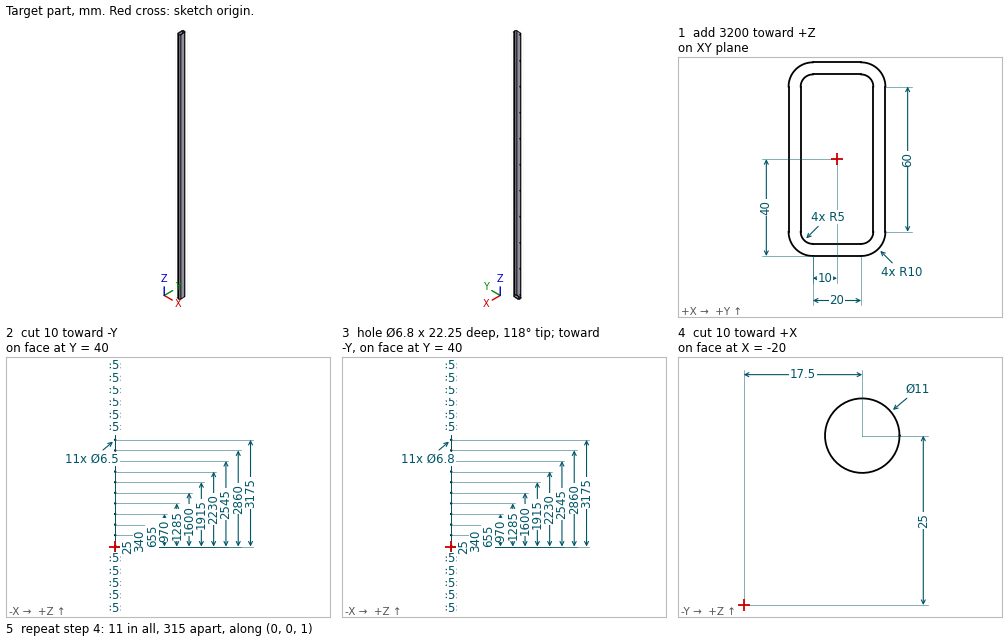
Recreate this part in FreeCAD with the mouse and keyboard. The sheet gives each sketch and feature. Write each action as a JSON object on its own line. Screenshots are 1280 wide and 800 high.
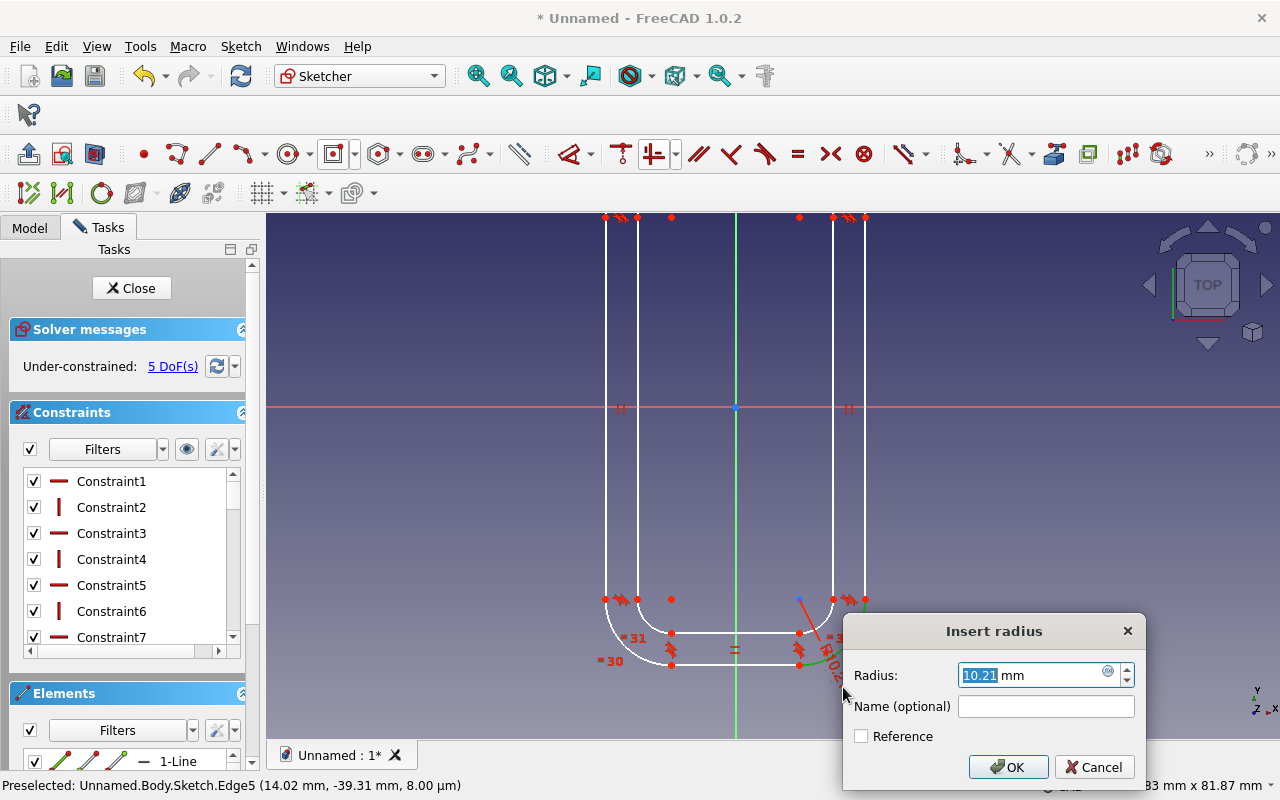
{"action": "type", "text": "10"}
{"action": "key", "text": "Return"}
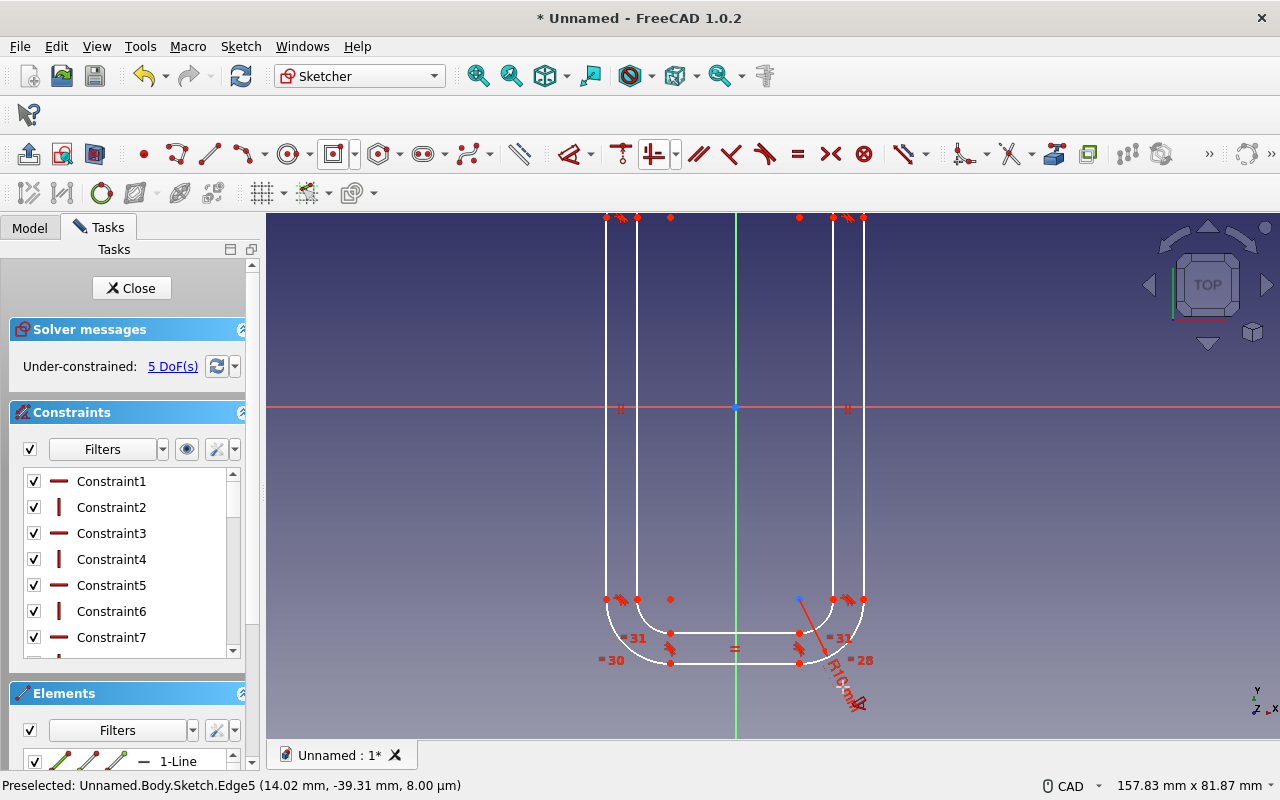
{"action": "scroll", "coordinate": [641, 615], "scroll_direction": "up", "scroll_amount": 2}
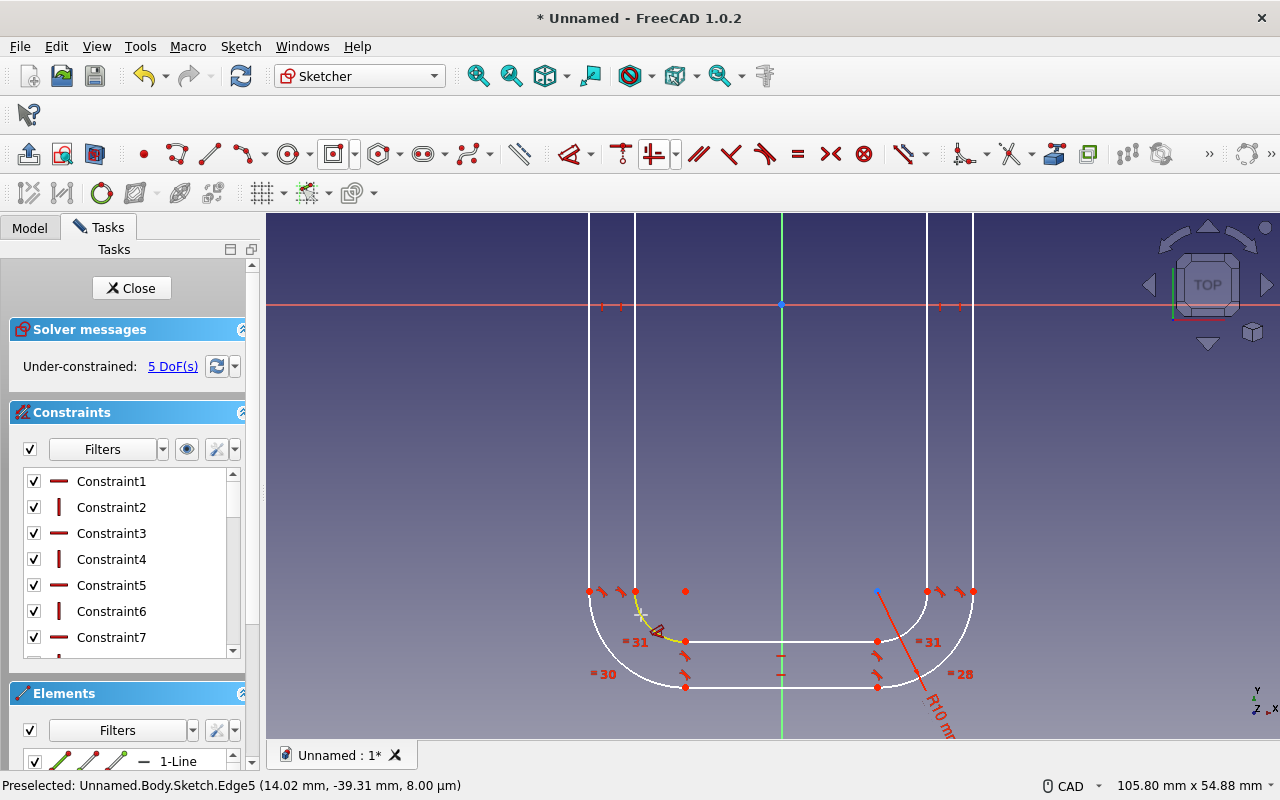
{"action": "left_click", "coordinate": [640, 615]}
{"action": "left_click", "coordinate": [612, 630]}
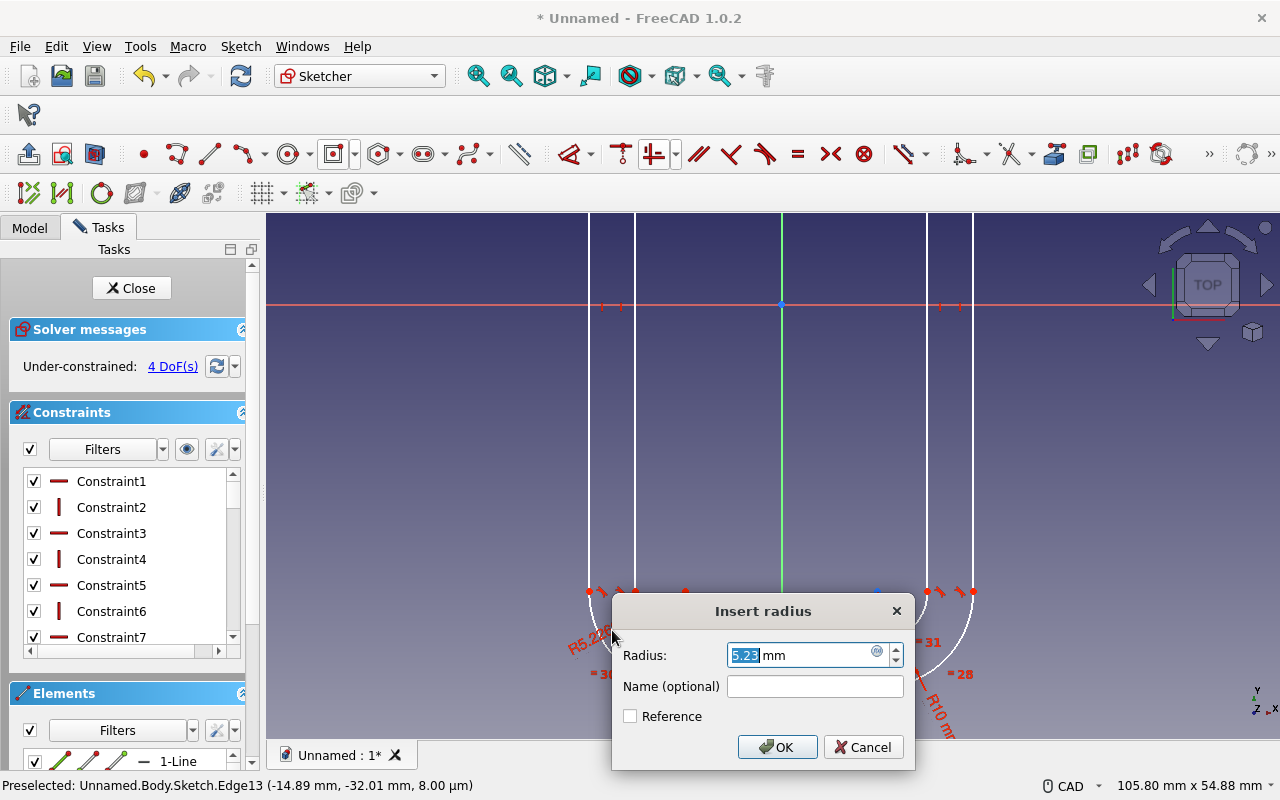
{"action": "type", "text": "5"}
{"action": "key", "text": "Return"}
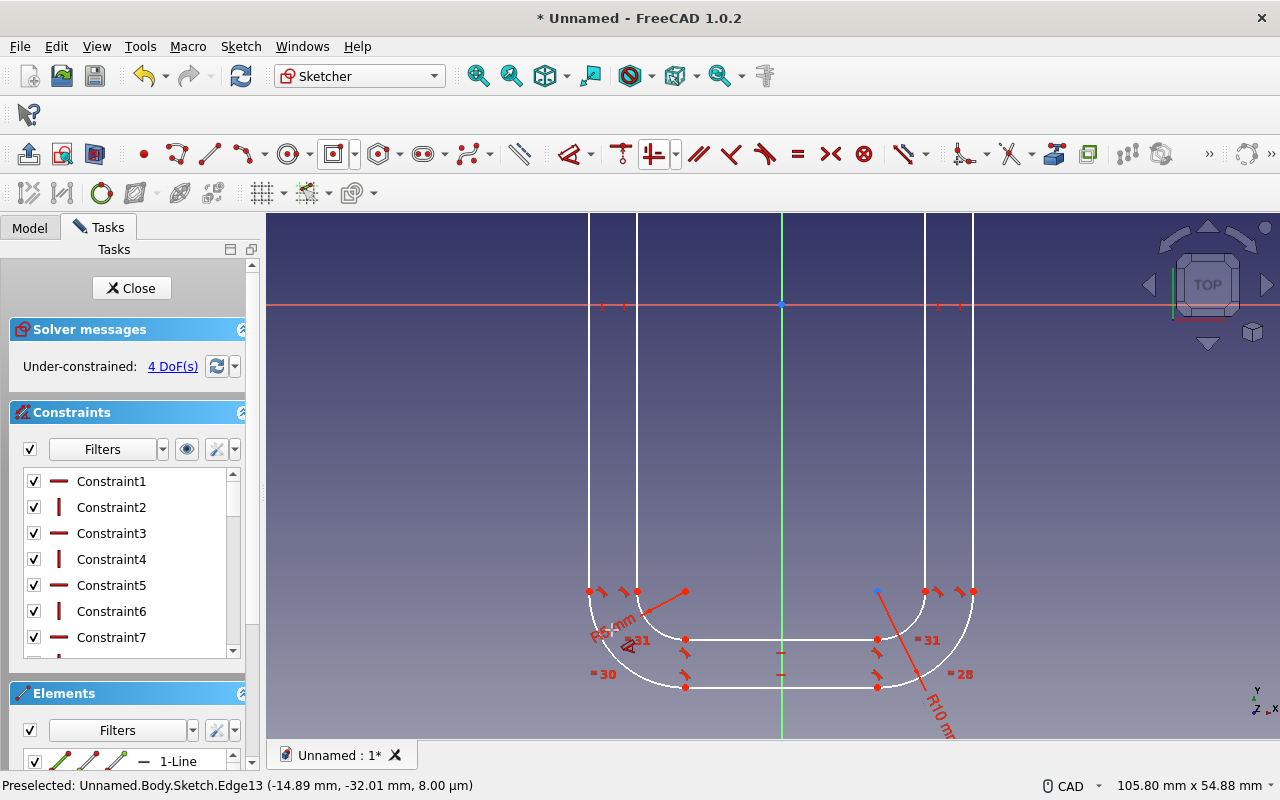
{"action": "left_click", "coordinate": [743, 688]}
{"action": "left_click", "coordinate": [737, 654]}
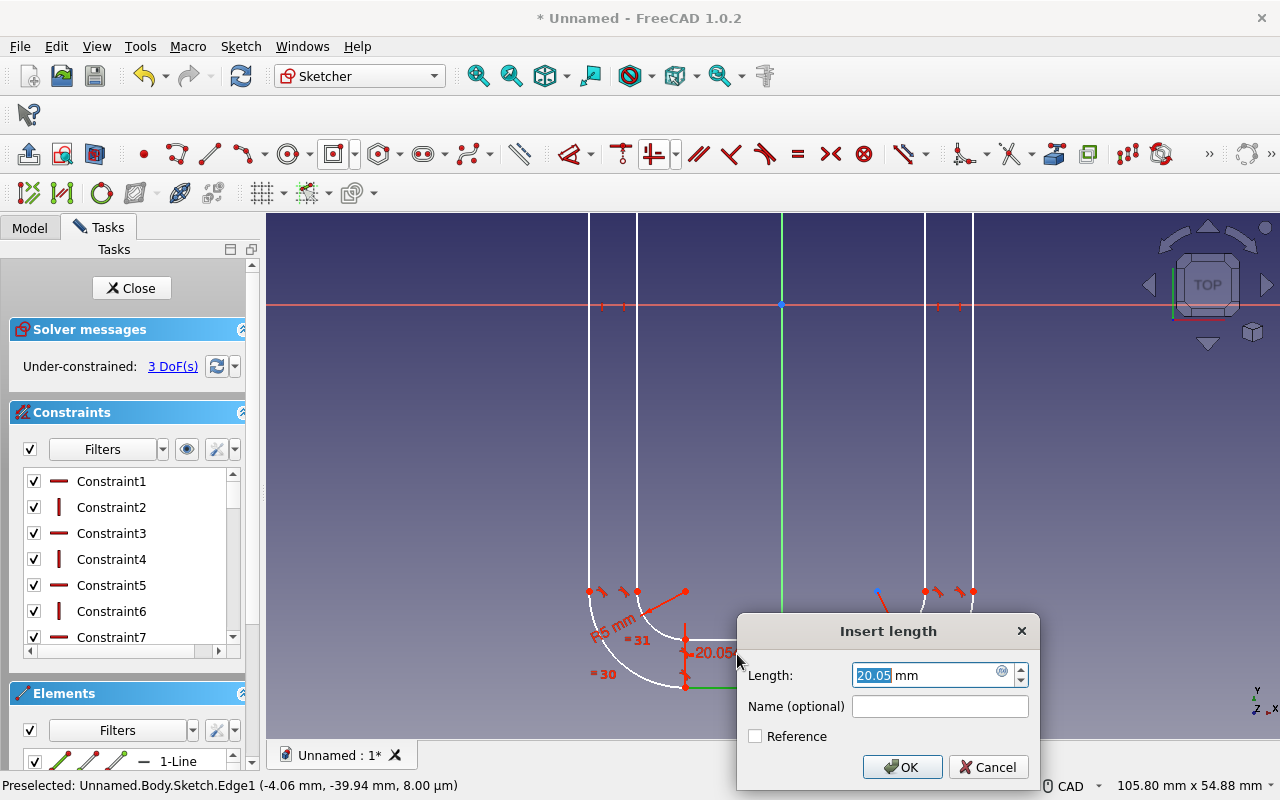
{"action": "type", "text": "20"}
{"action": "key", "text": "Return"}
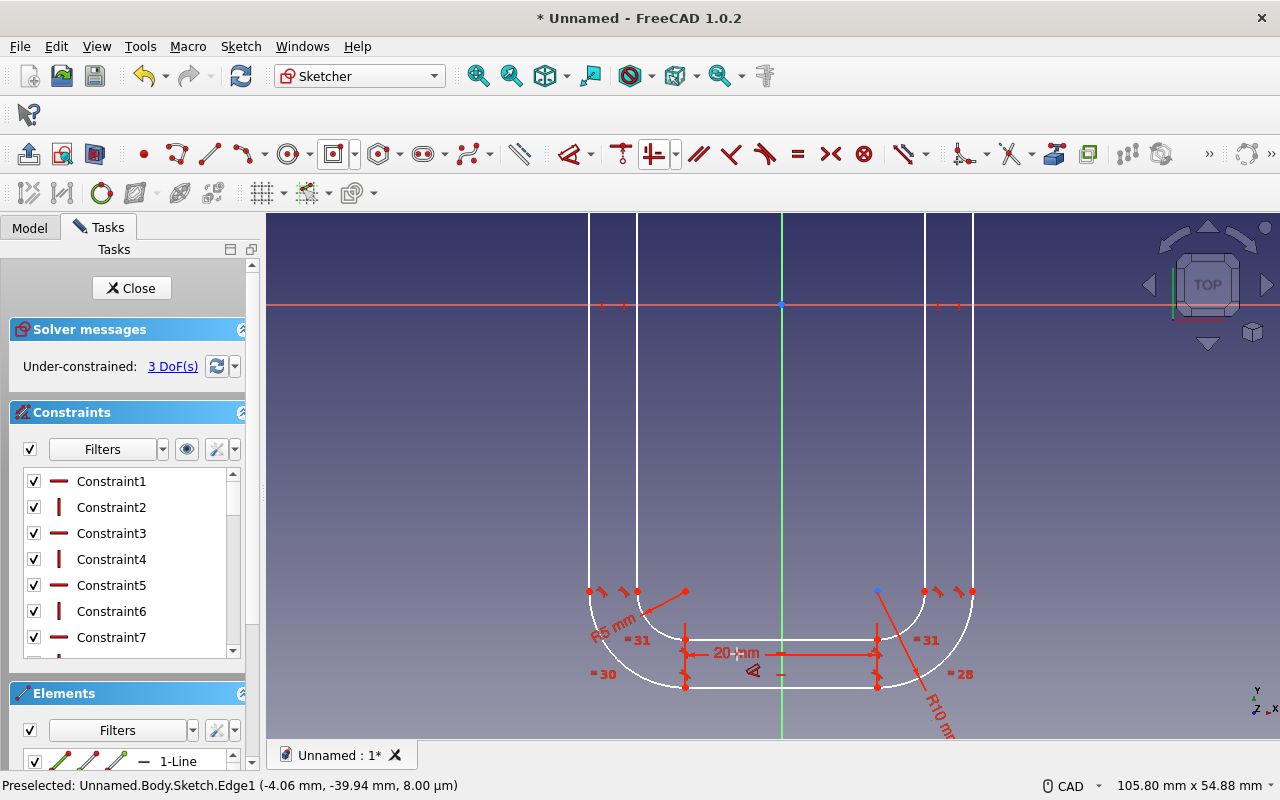
{"action": "left_click", "coordinate": [973, 421]}
{"action": "left_click", "coordinate": [1007, 416]}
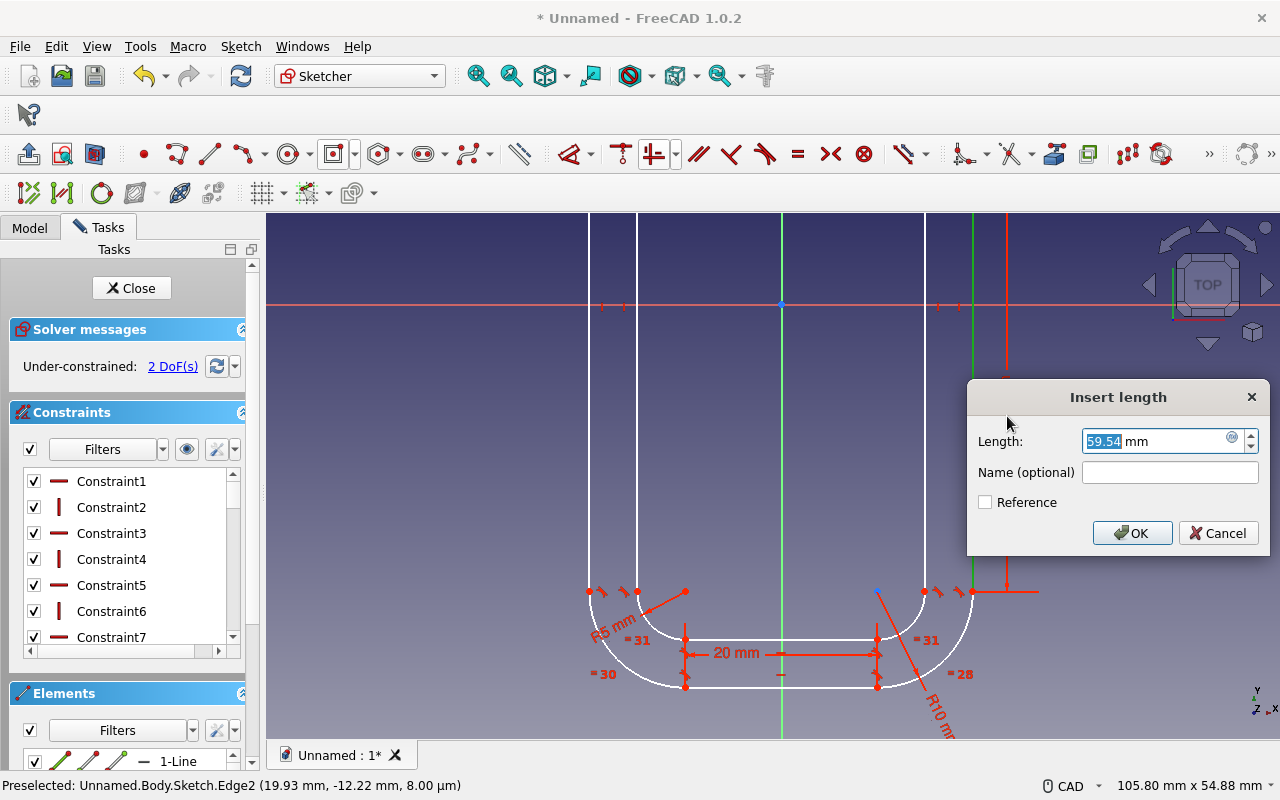
{"action": "type", "text": "60"}
{"action": "key", "text": "Return"}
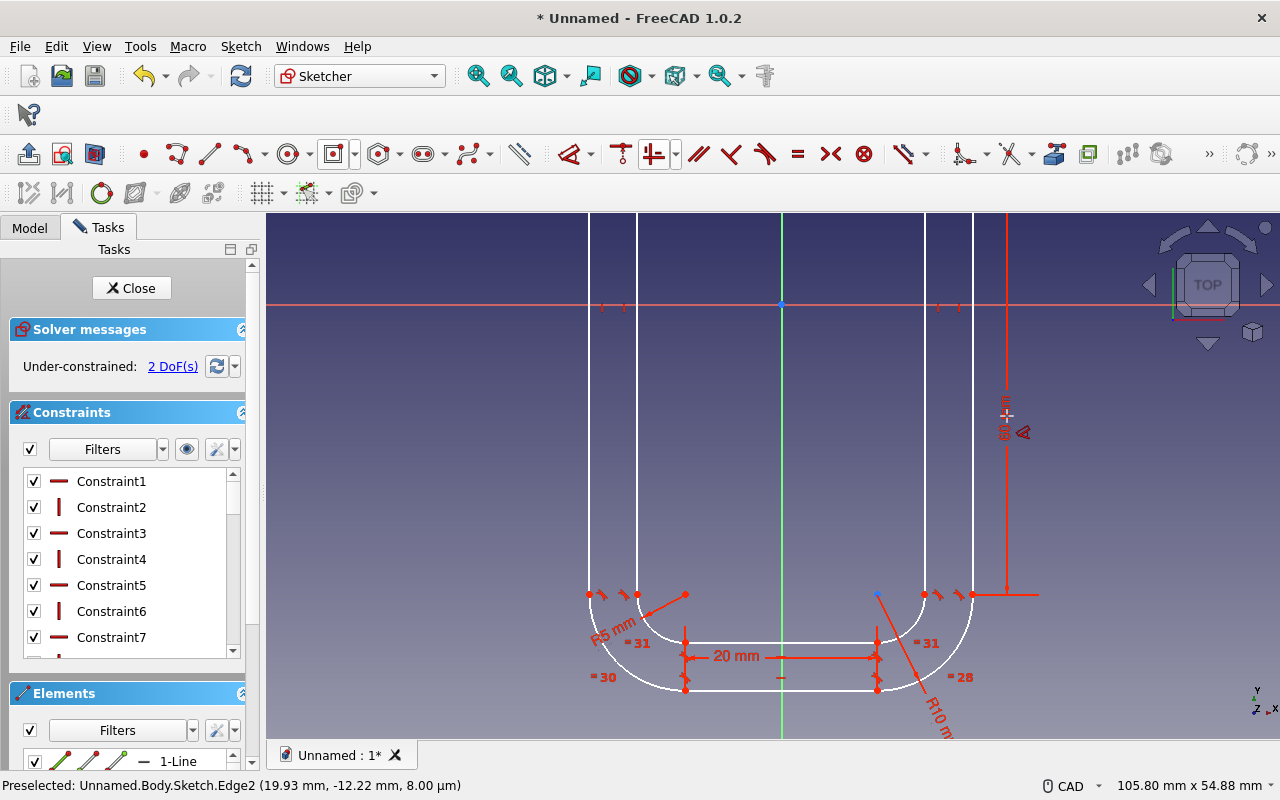
{"action": "left_click", "coordinate": [685, 691]}
{"action": "left_click", "coordinate": [734, 271]}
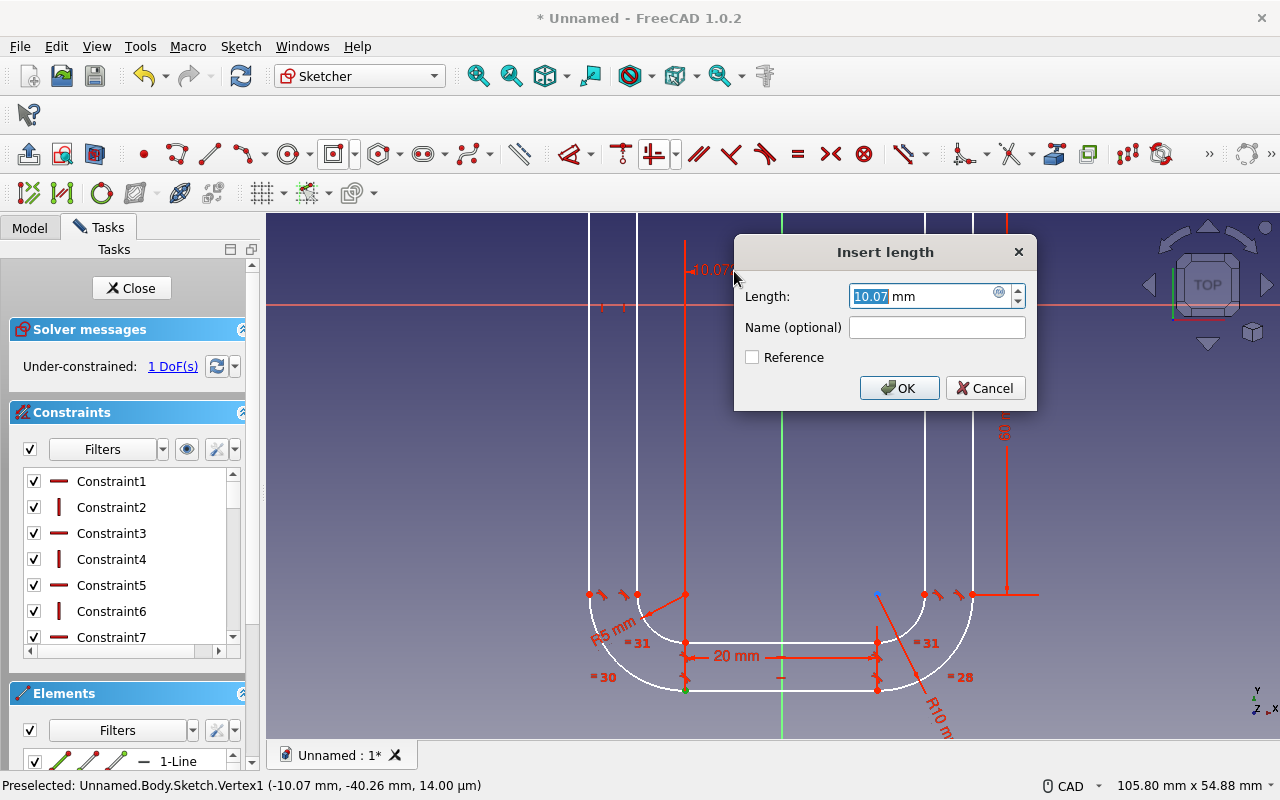
{"action": "type", "text": "10"}
{"action": "key", "text": "Return"}